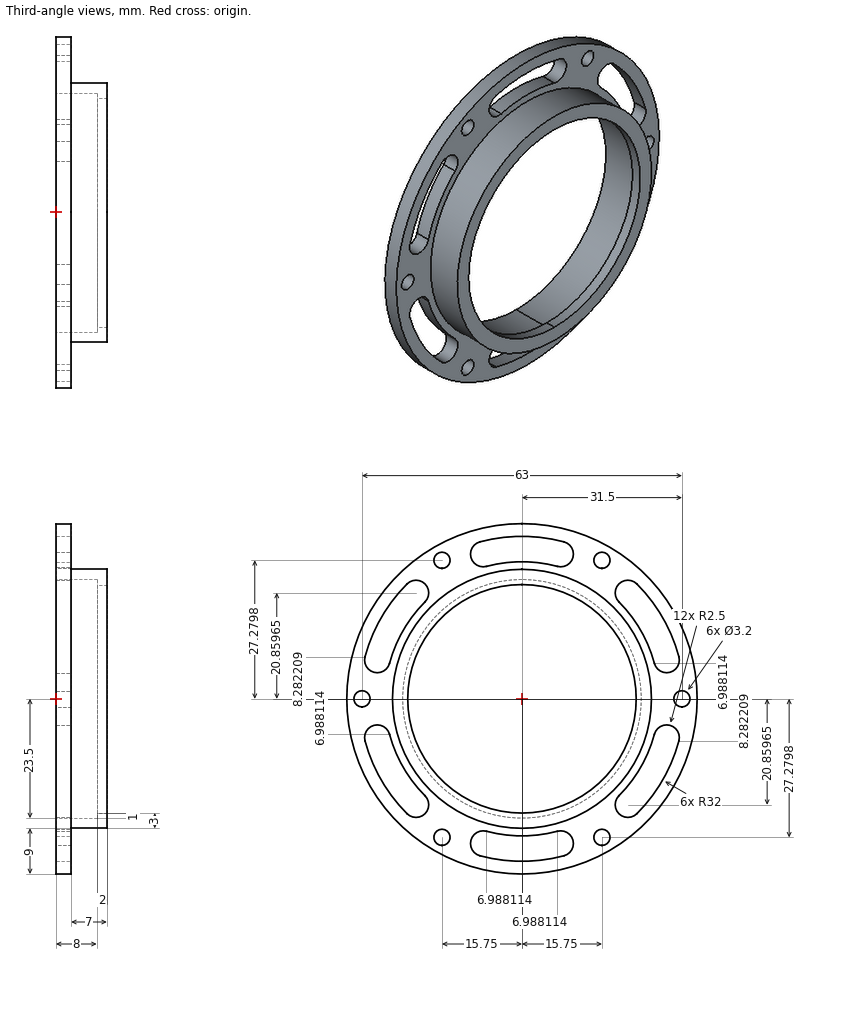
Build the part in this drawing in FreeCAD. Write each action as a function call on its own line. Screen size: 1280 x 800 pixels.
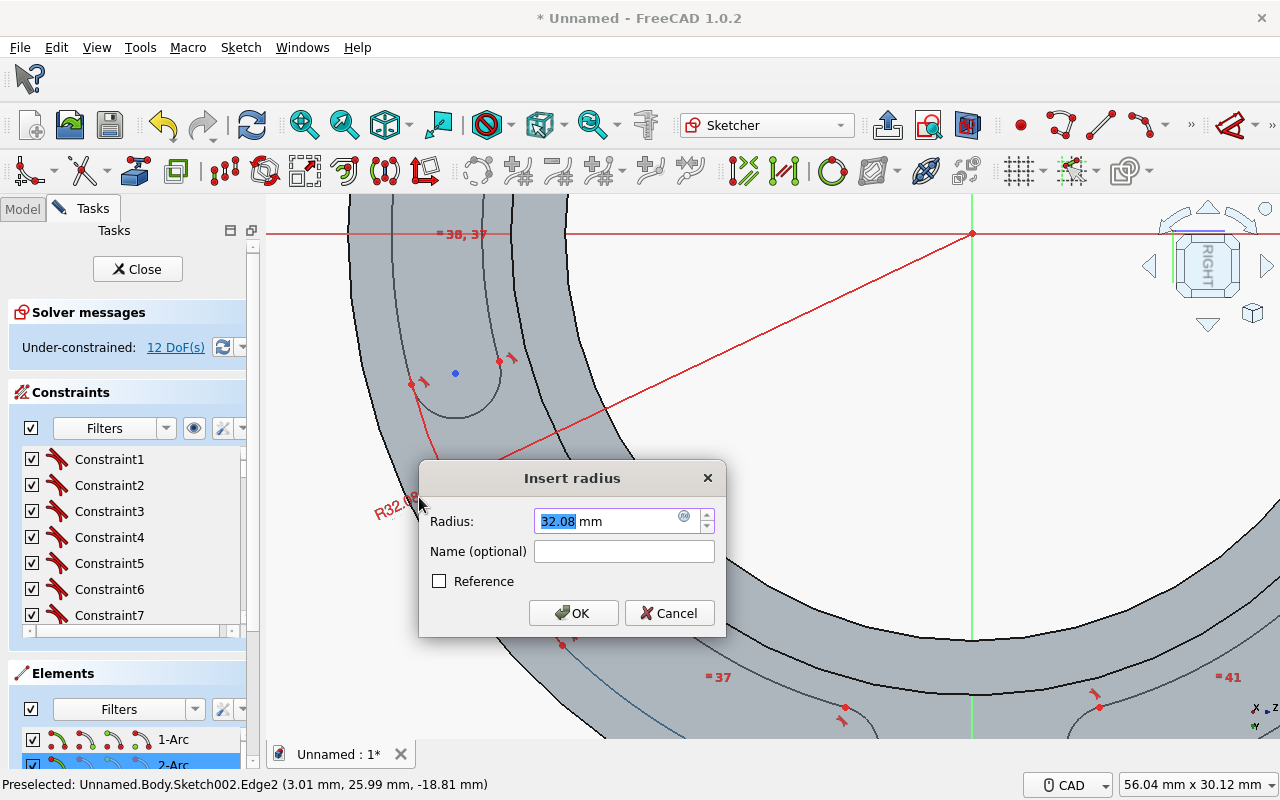
text(32)
key(Return)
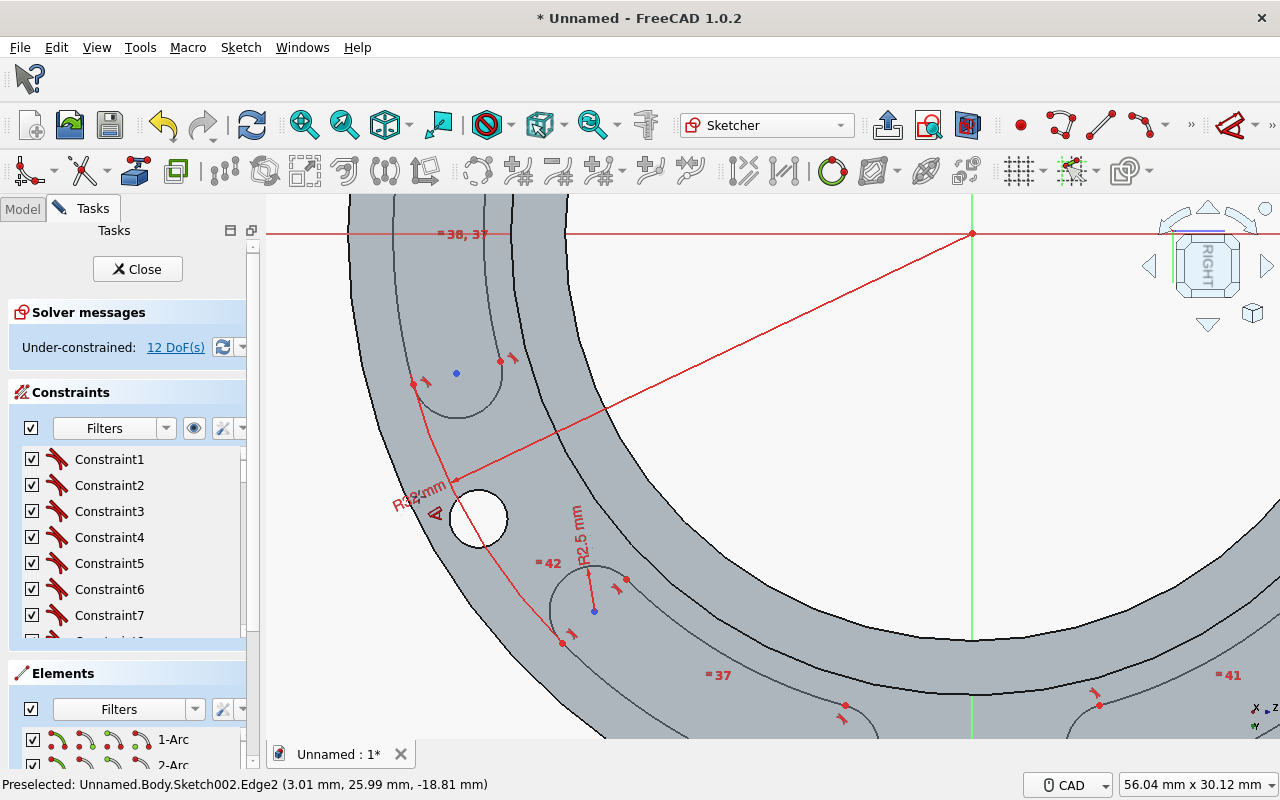
scroll(589, 567, down, 6)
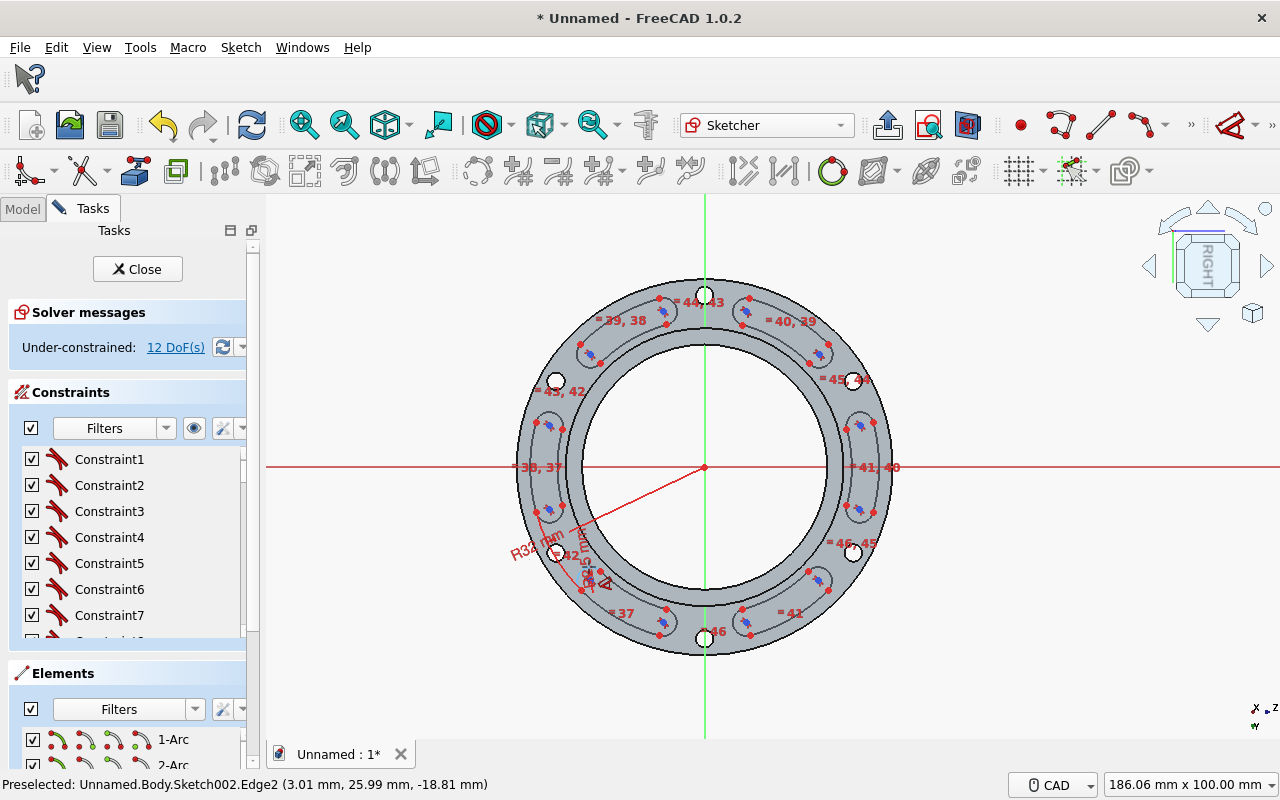
click(660, 636)
click(682, 670)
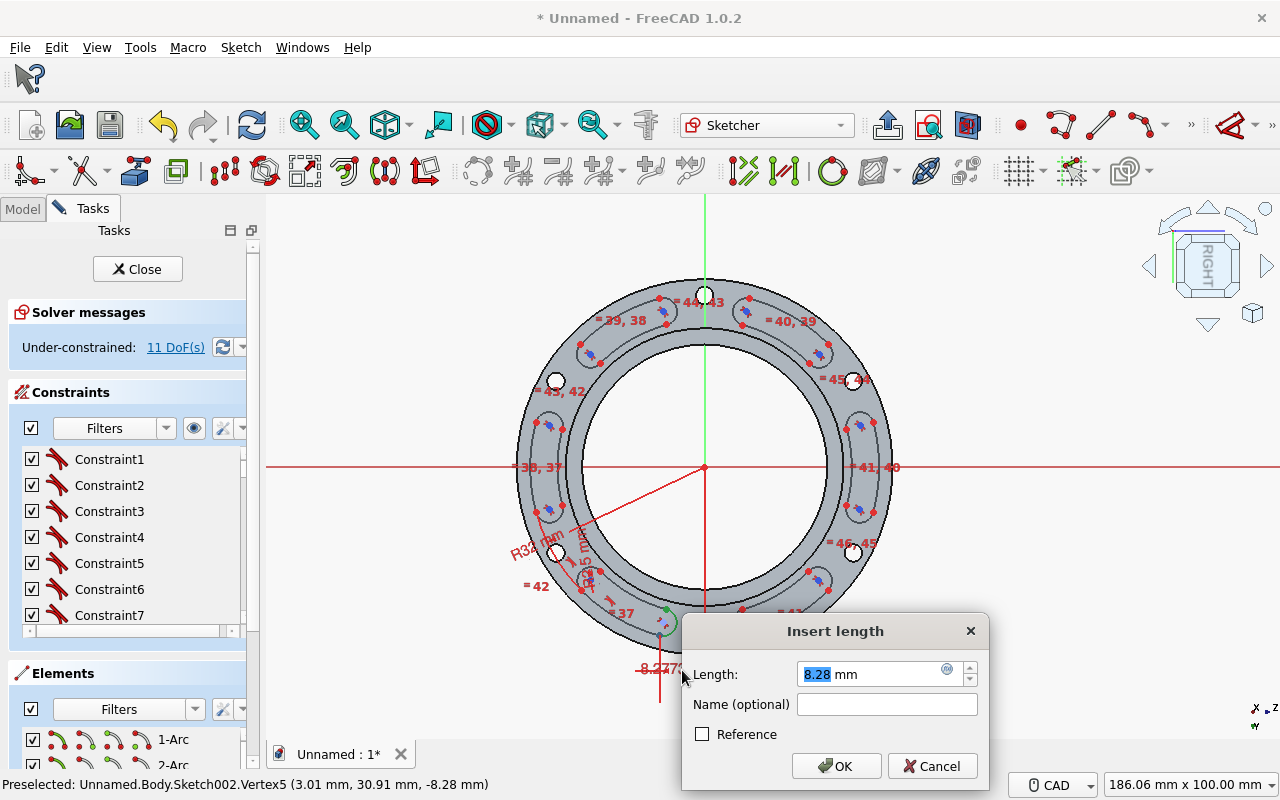
text(8.282209)
key(Return)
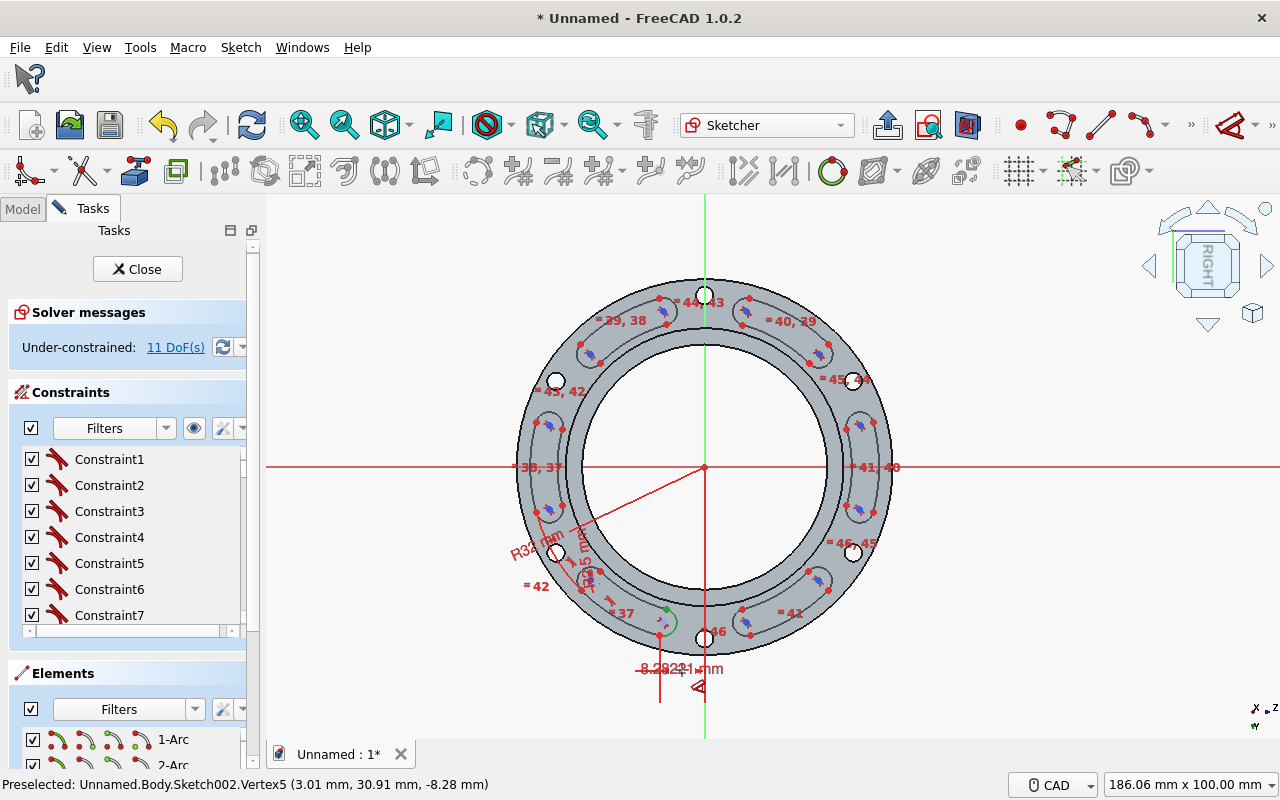
click(562, 429)
click(739, 448)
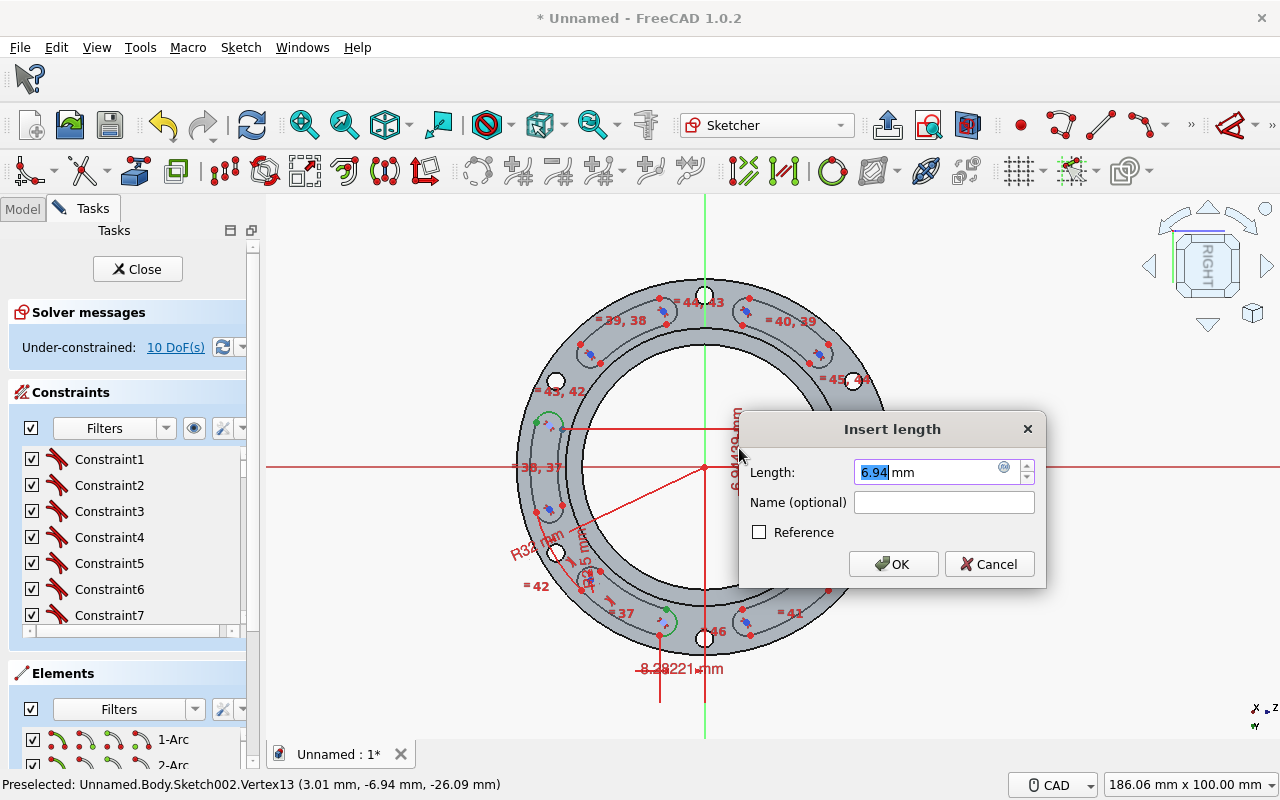
text(6.988114)
key(Return)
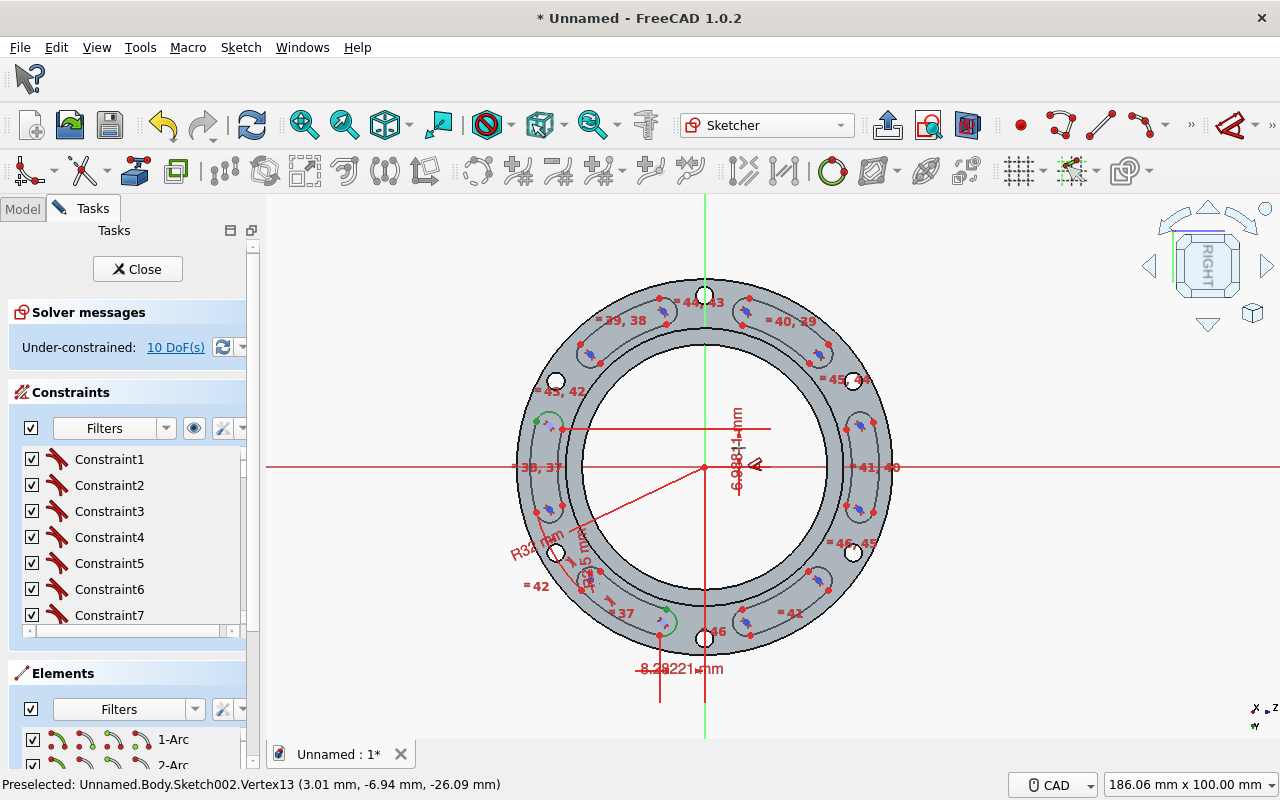
click(563, 506)
click(739, 486)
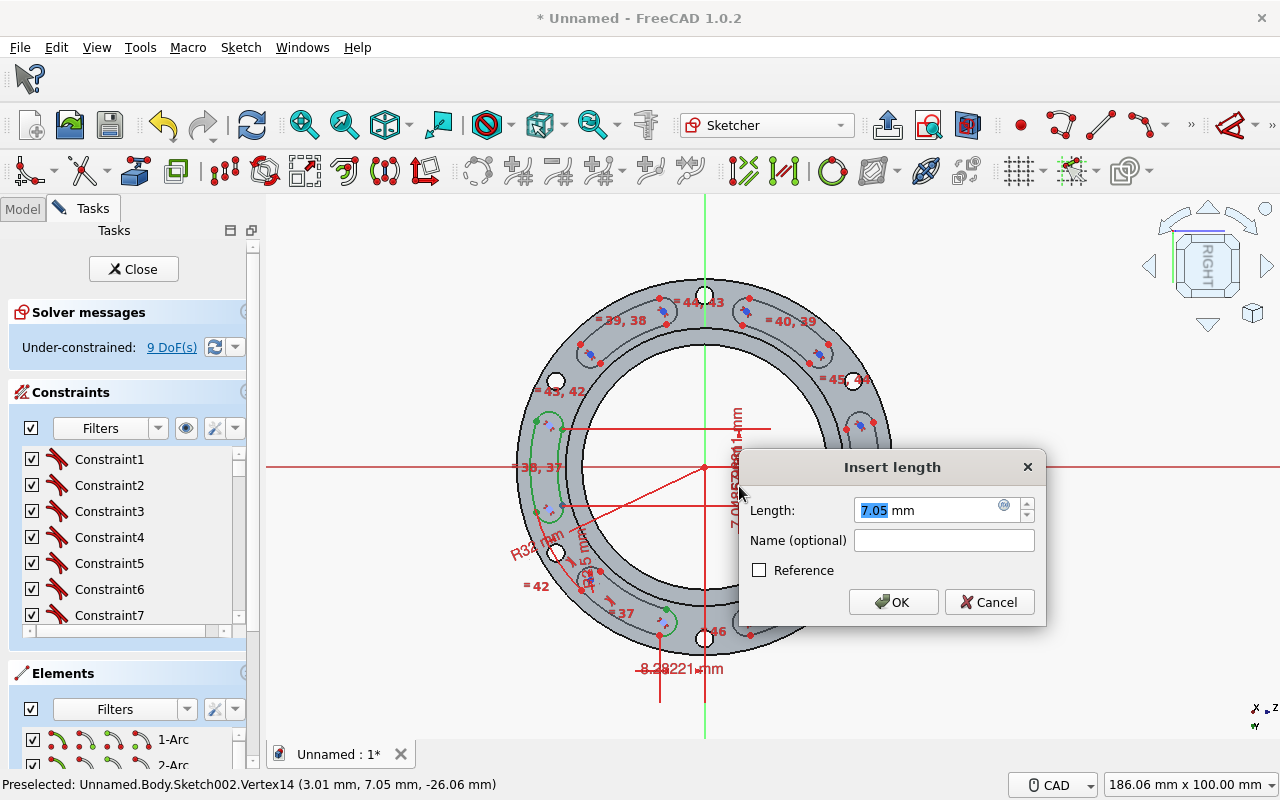
text(6.988114)
key(Return)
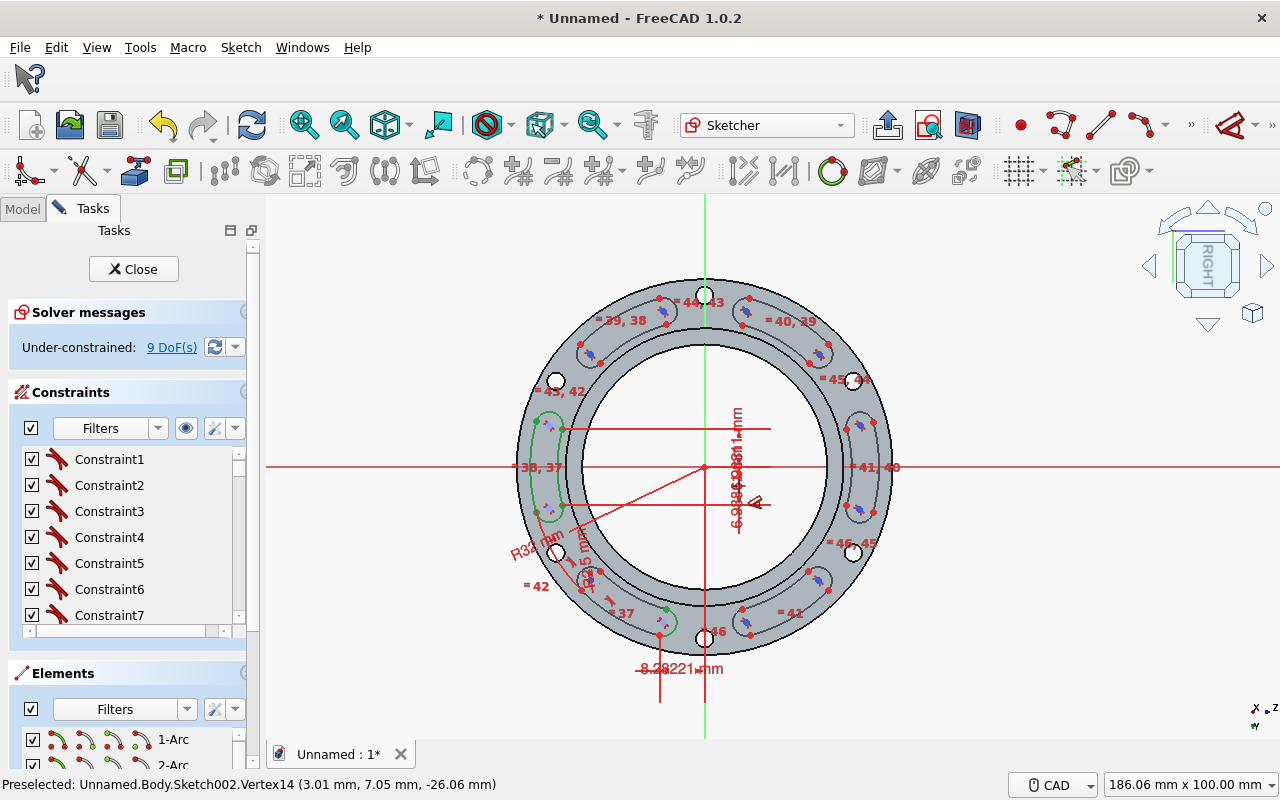
click(667, 325)
click(686, 291)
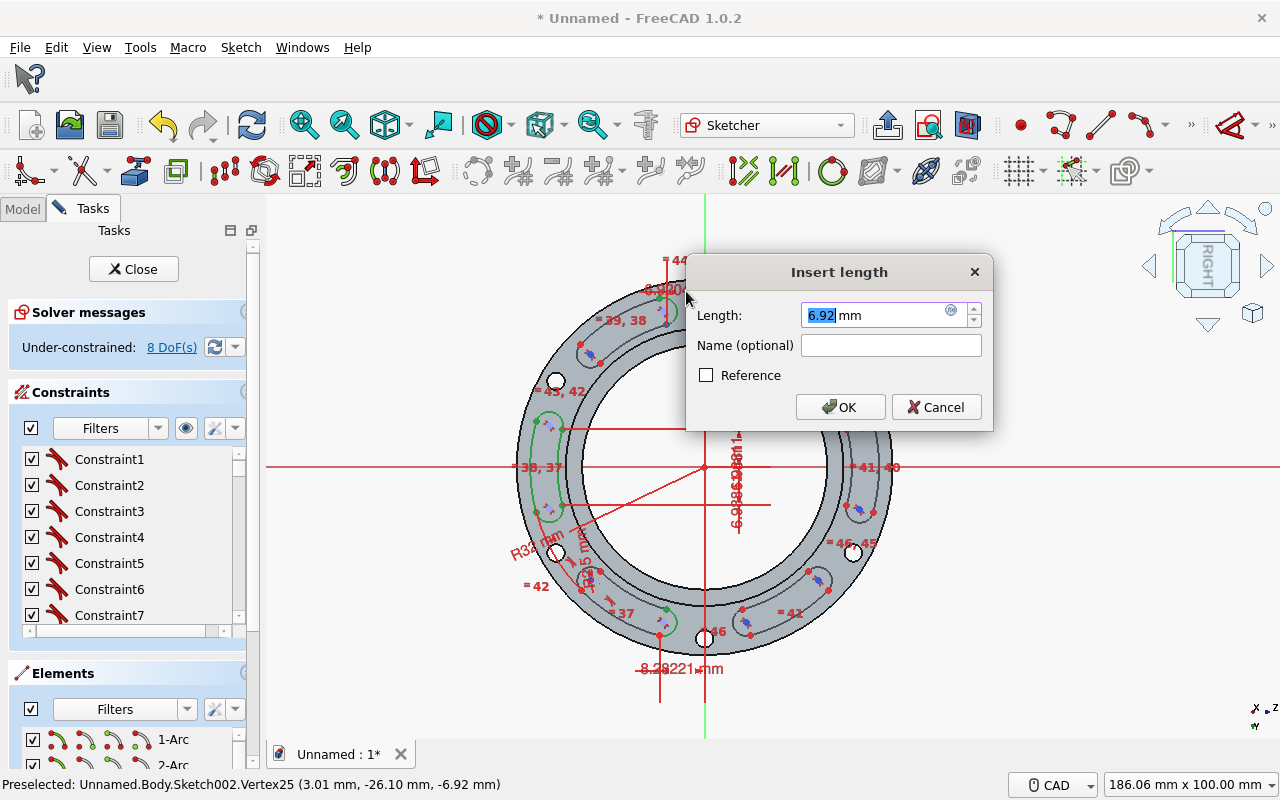
text(6.988114)
key(Return)